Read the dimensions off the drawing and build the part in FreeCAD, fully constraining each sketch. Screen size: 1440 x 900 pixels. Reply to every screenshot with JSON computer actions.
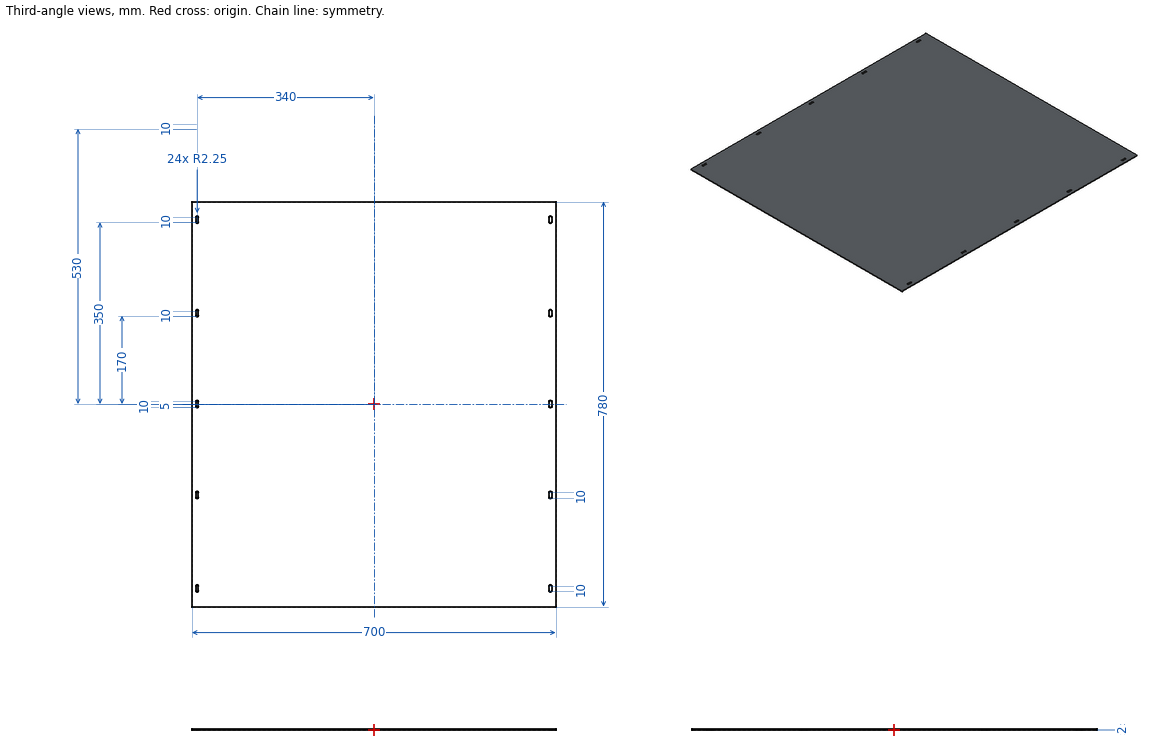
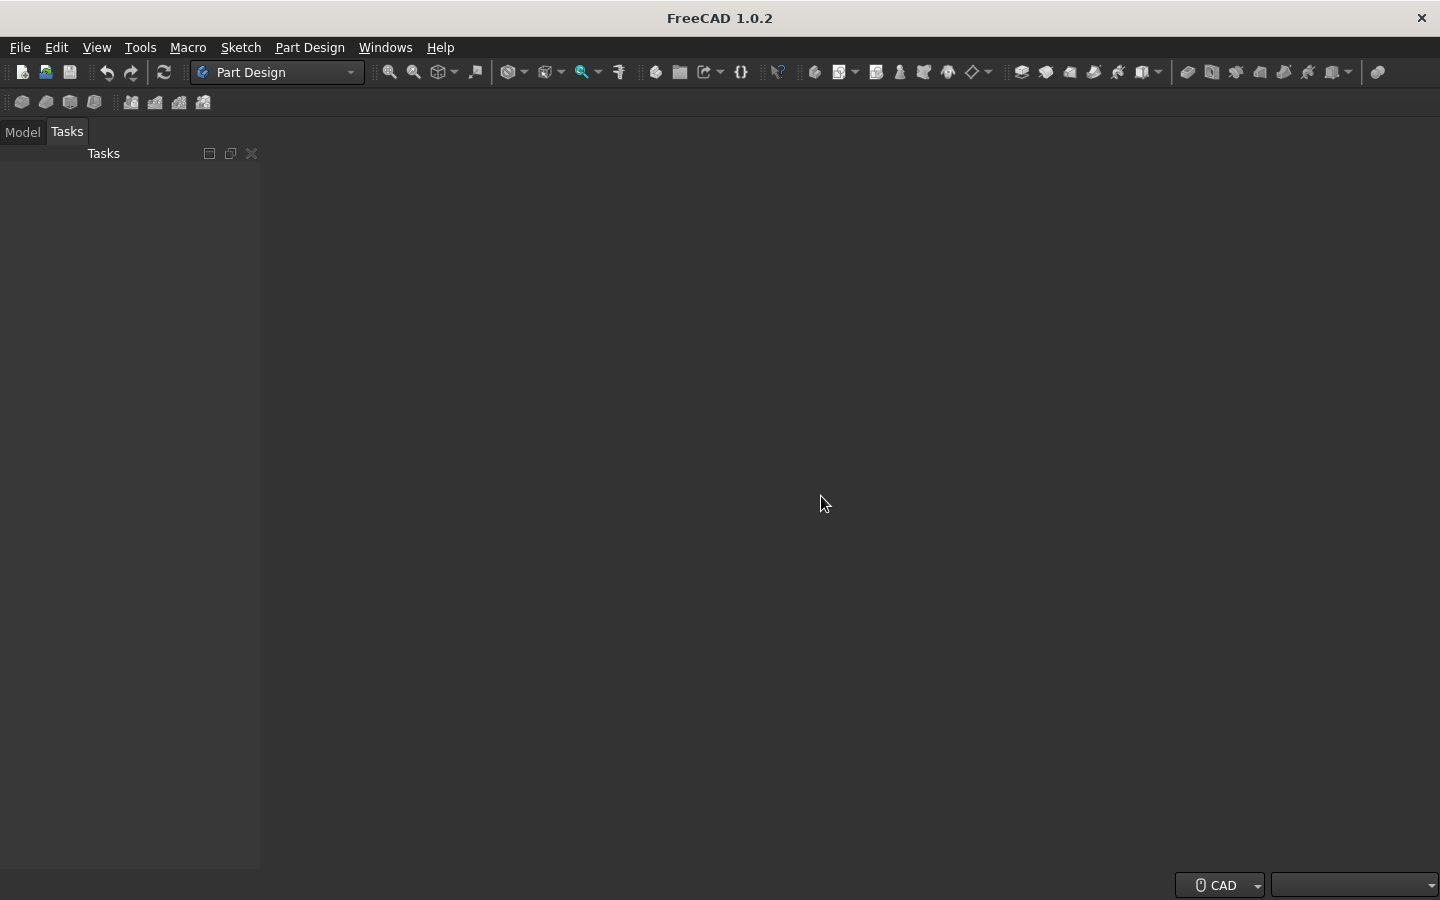
{"action": "key", "text": "ctrl+n"}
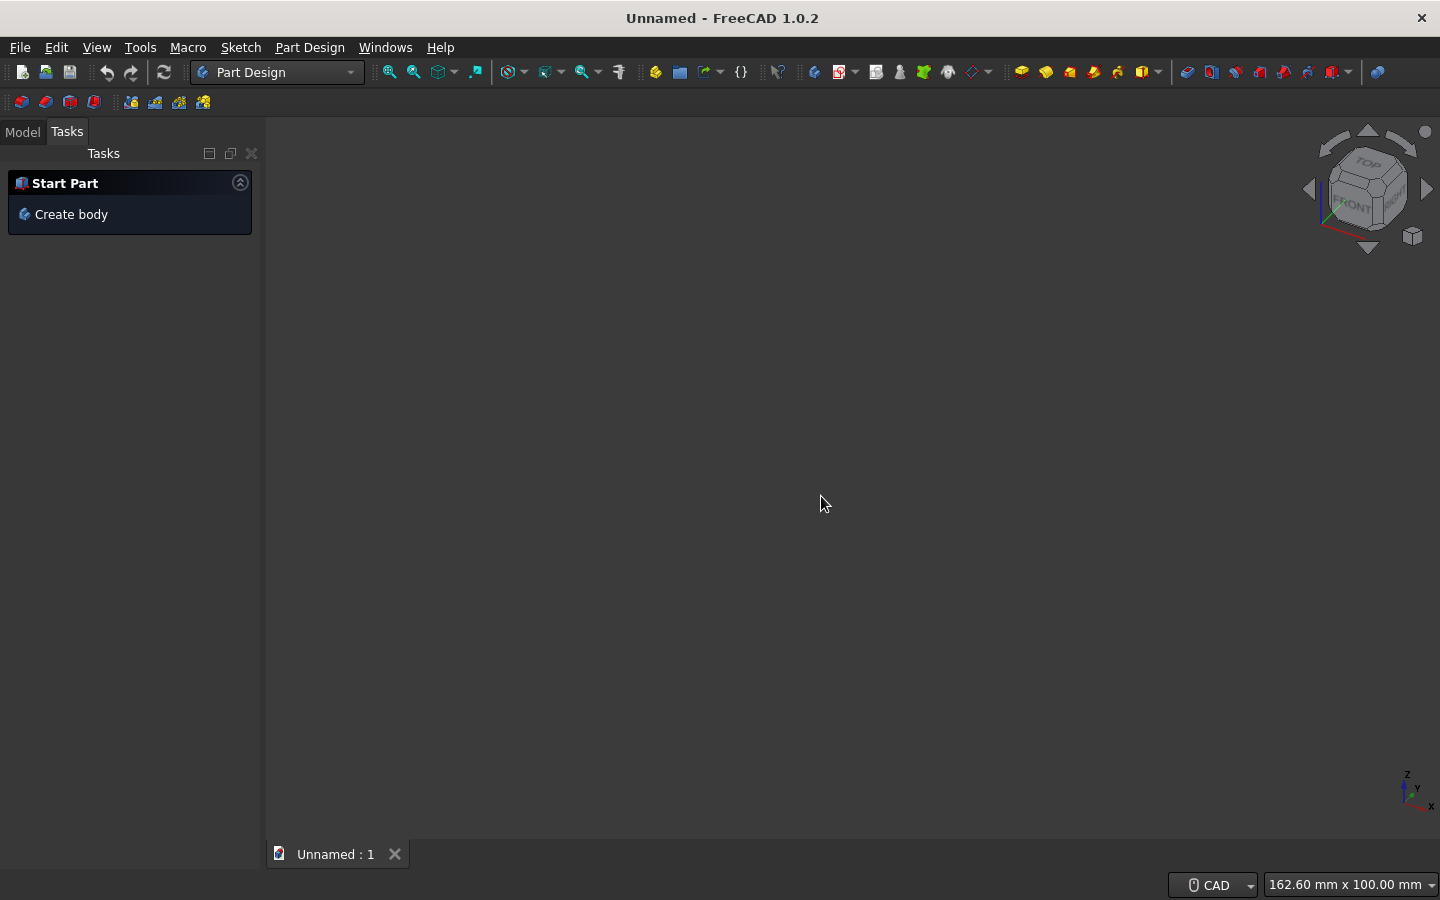
{"action": "left_click", "coordinate": [840, 72]}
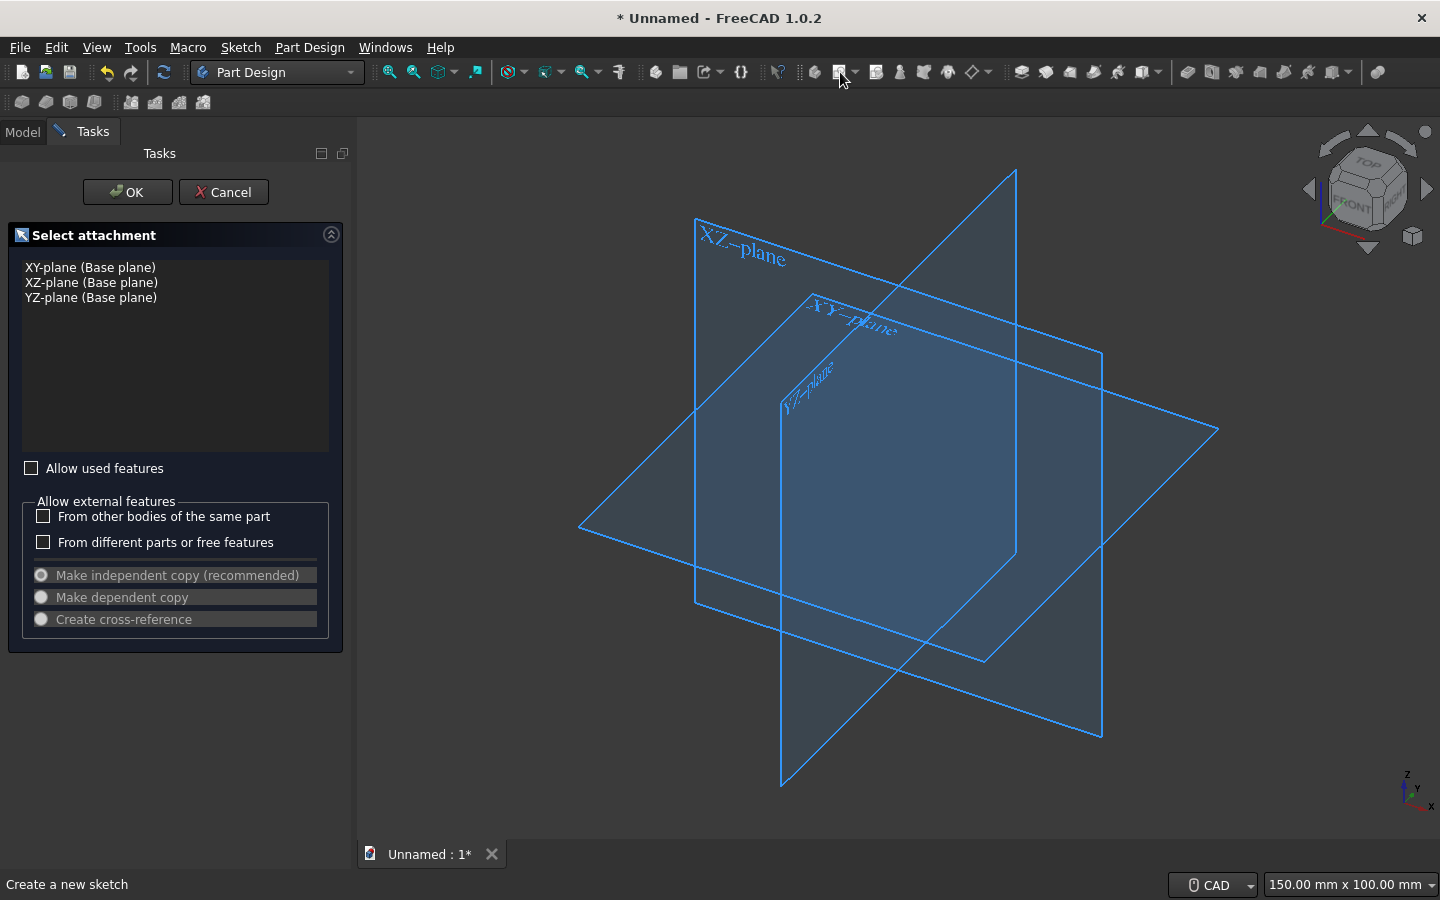
{"action": "left_click", "coordinate": [82, 268]}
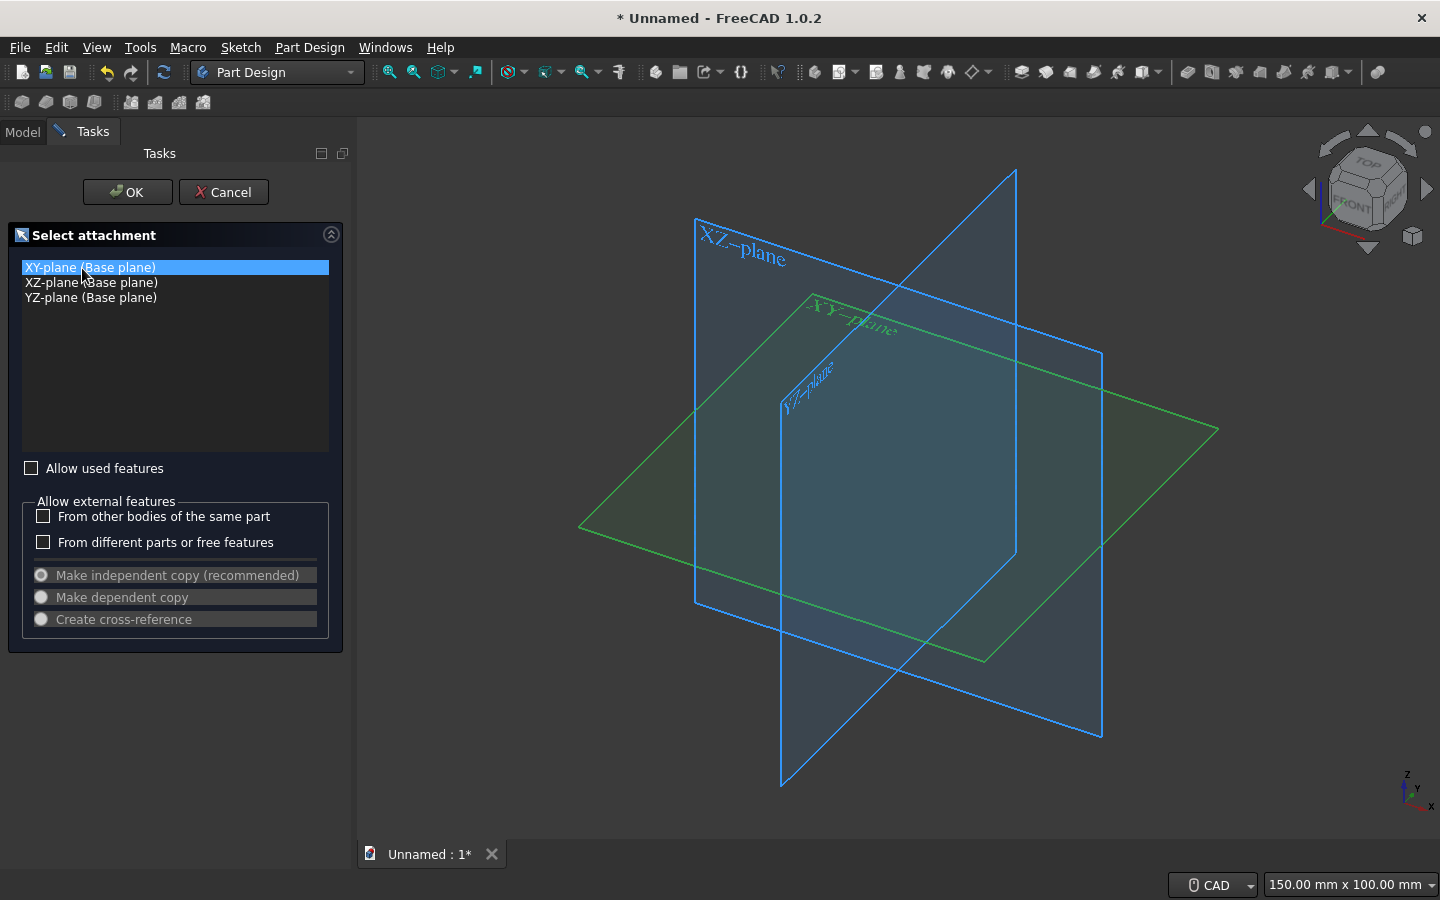
{"action": "left_click", "coordinate": [128, 192]}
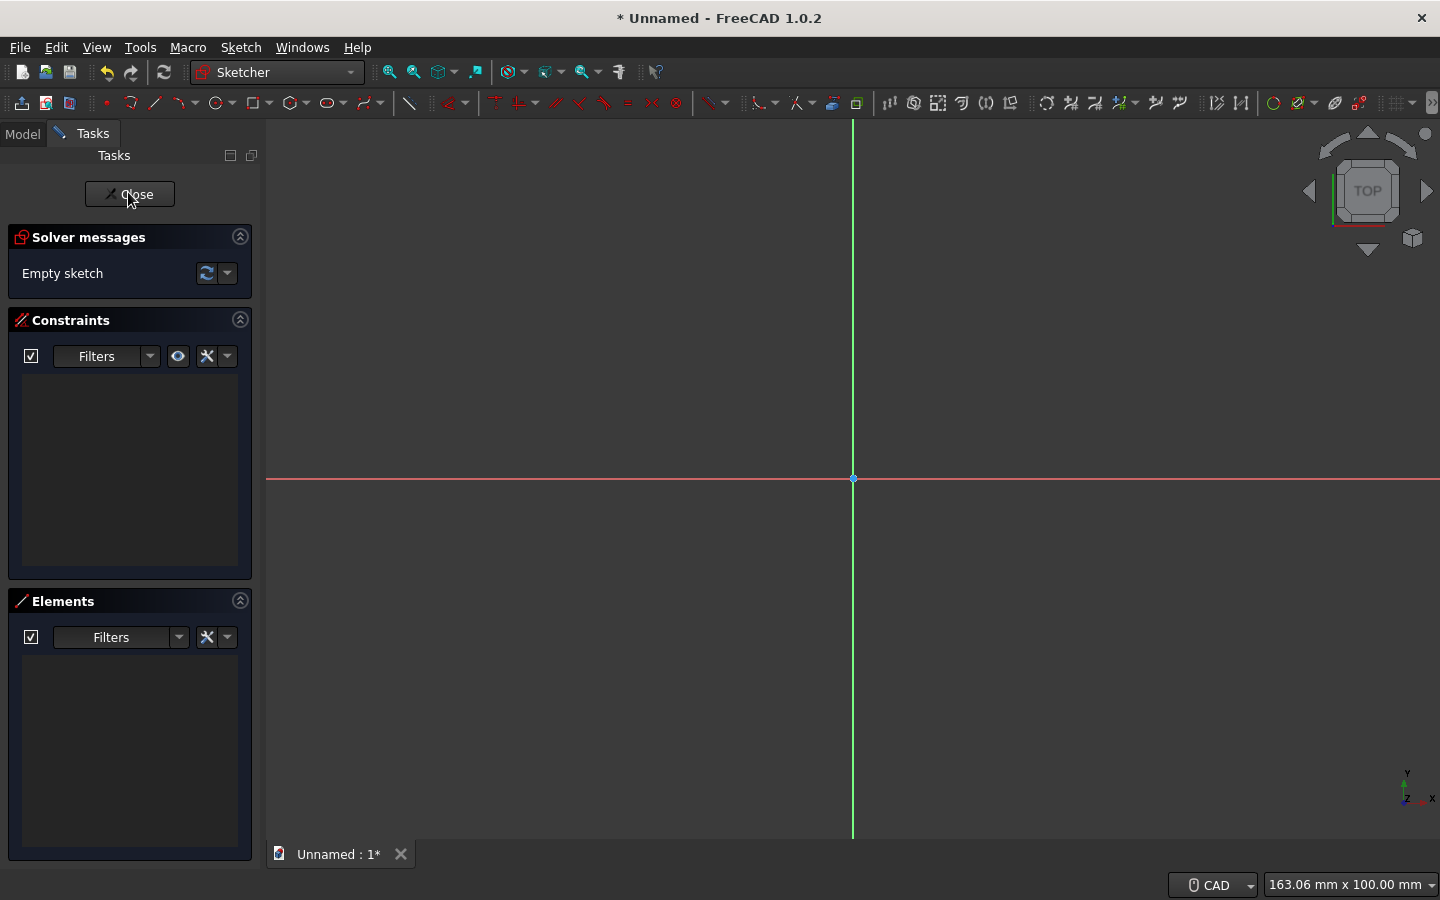
{"action": "scroll", "coordinate": [778, 479], "scroll_direction": "down", "scroll_amount": 12}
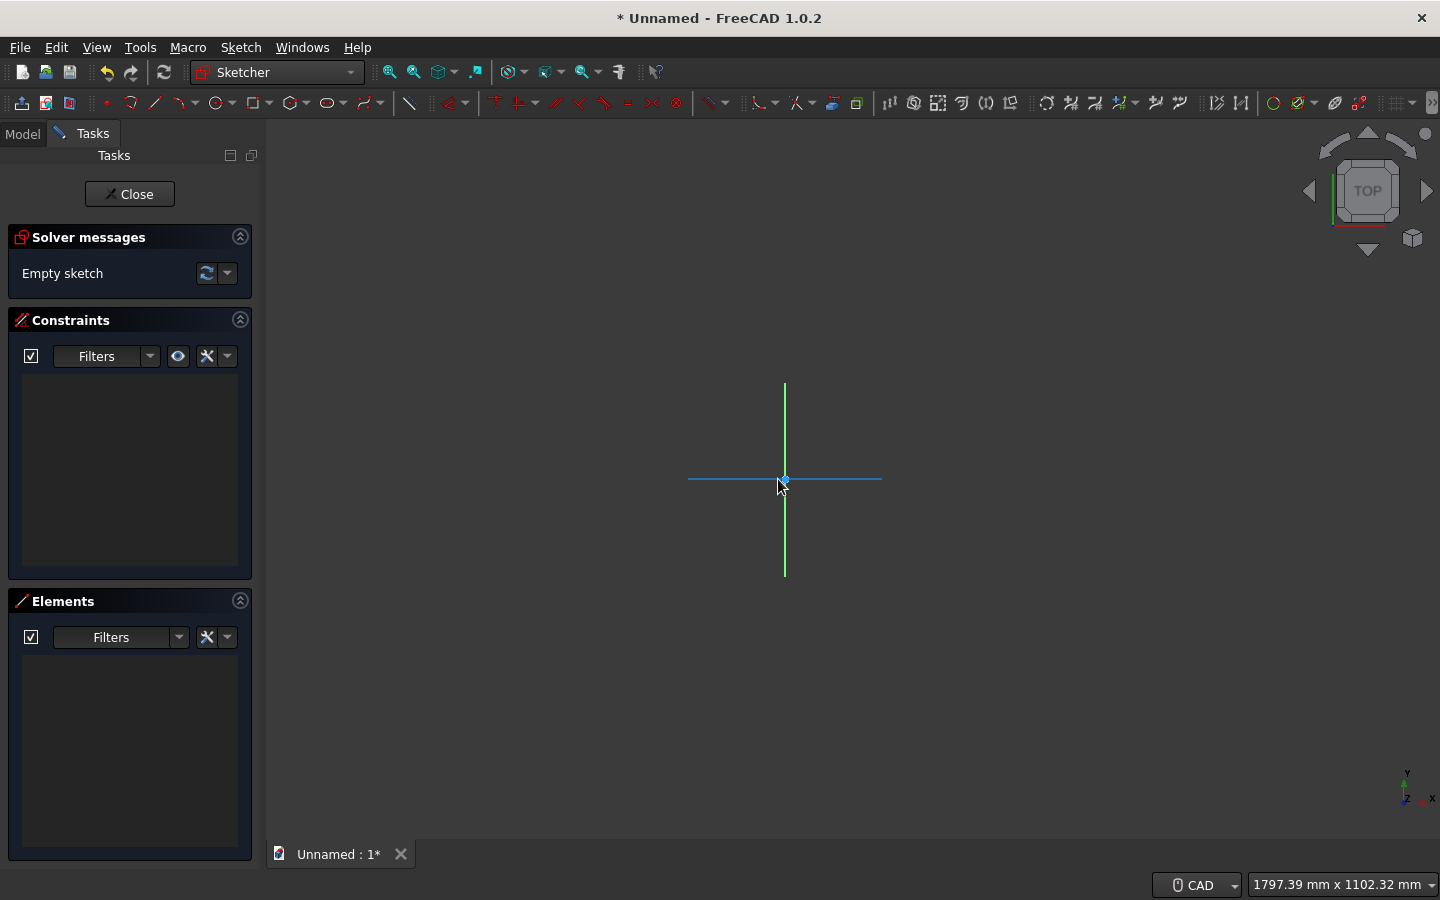
{"action": "key", "text": "g v"}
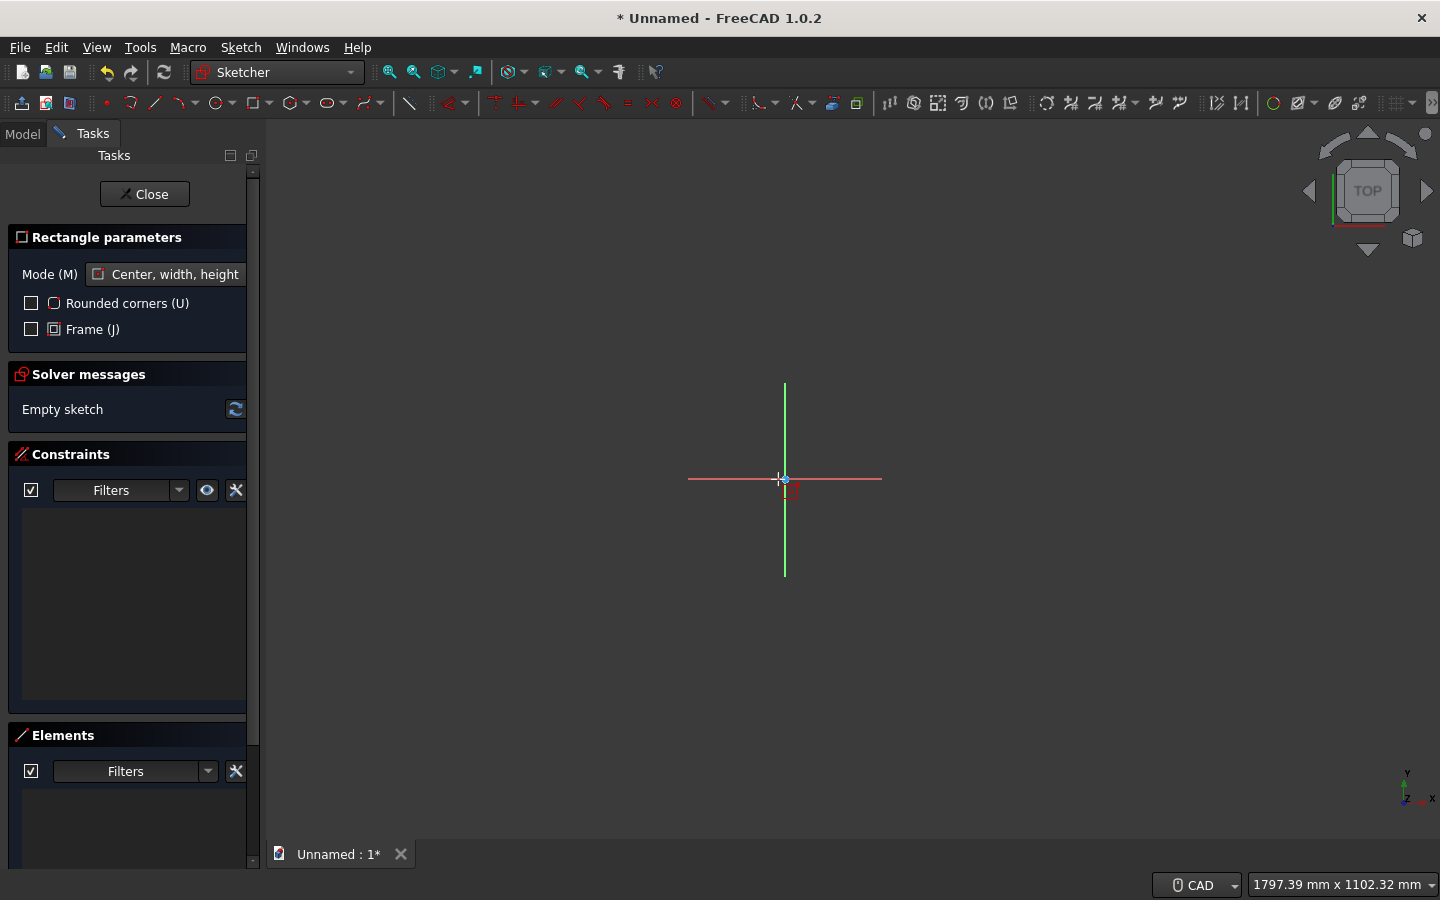
{"action": "left_click", "coordinate": [785, 479]}
{"action": "mouse_move", "coordinate": [1014, 225]}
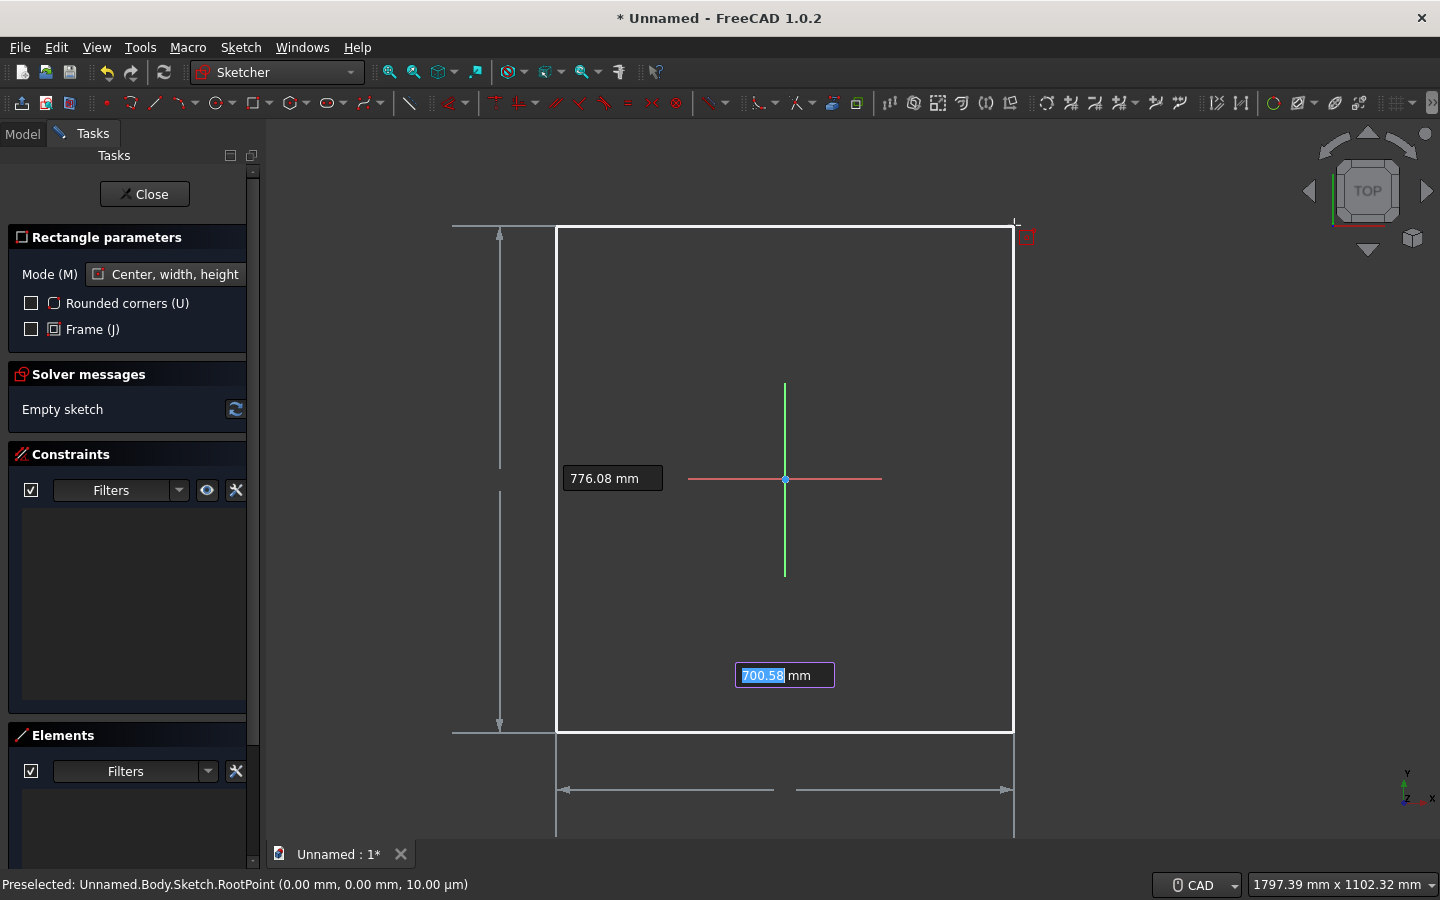
{"action": "type", "text": "700"}
{"action": "key", "text": "Tab"}
{"action": "type", "text": "780"}
{"action": "key", "text": "Return"}
{"action": "key", "text": "Escape"}